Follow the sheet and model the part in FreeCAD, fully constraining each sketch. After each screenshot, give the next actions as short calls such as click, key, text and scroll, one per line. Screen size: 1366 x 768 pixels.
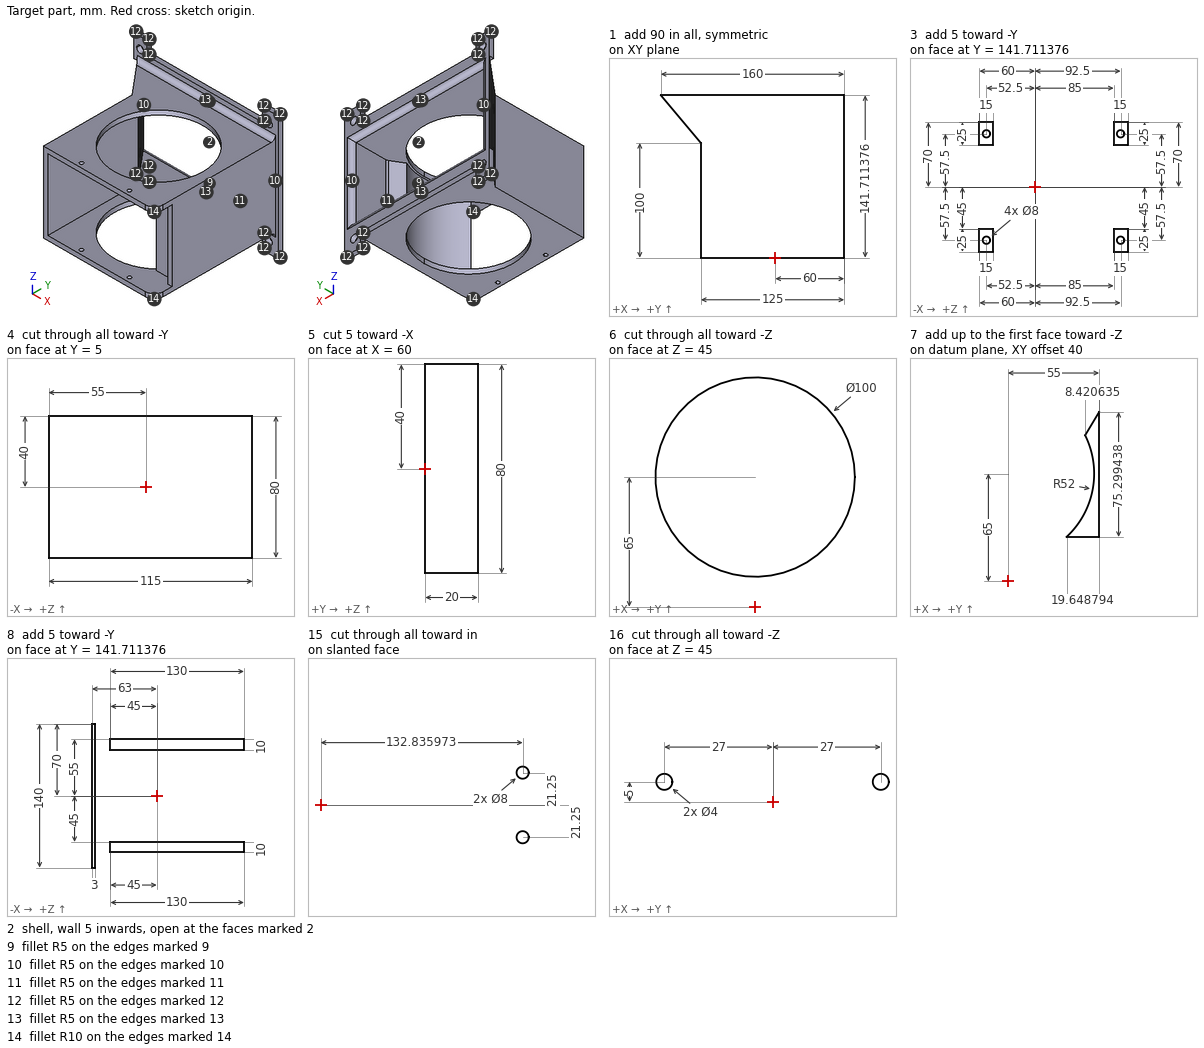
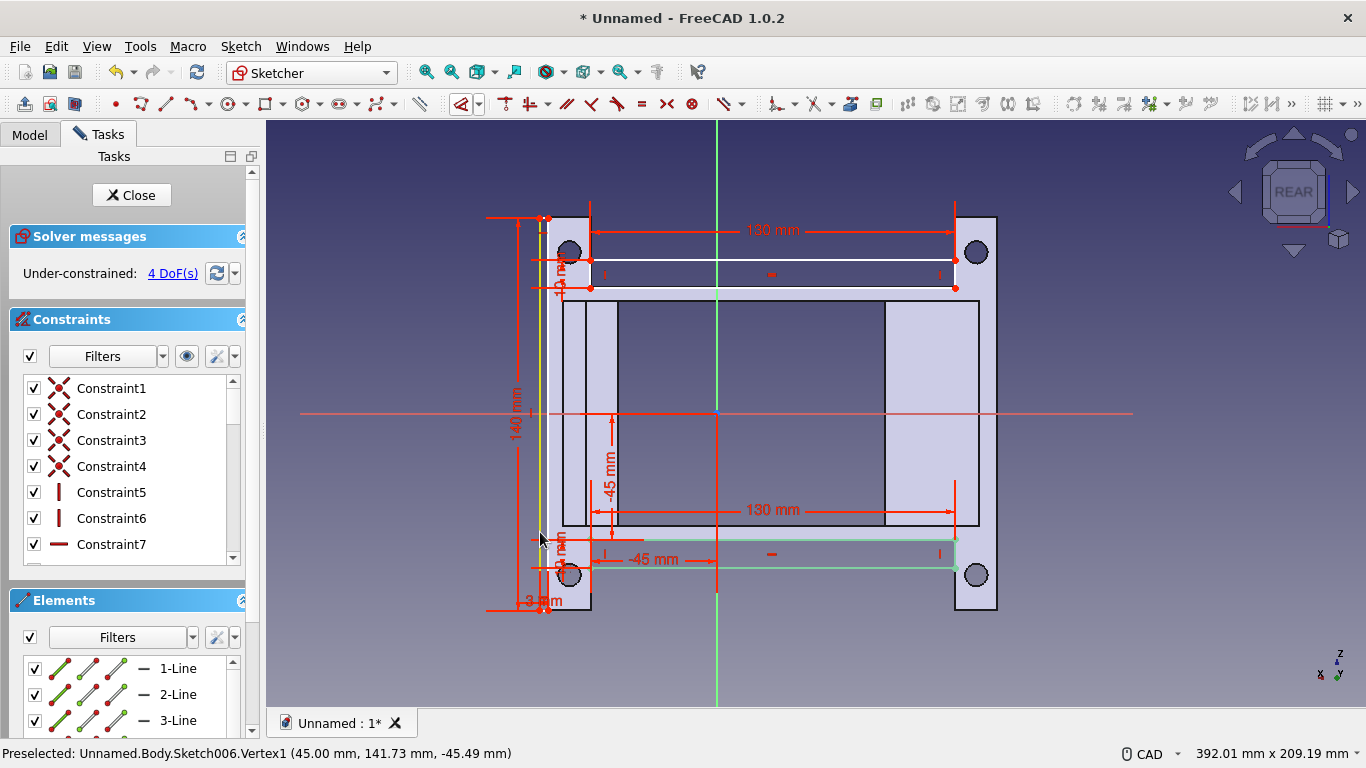
click(590, 260)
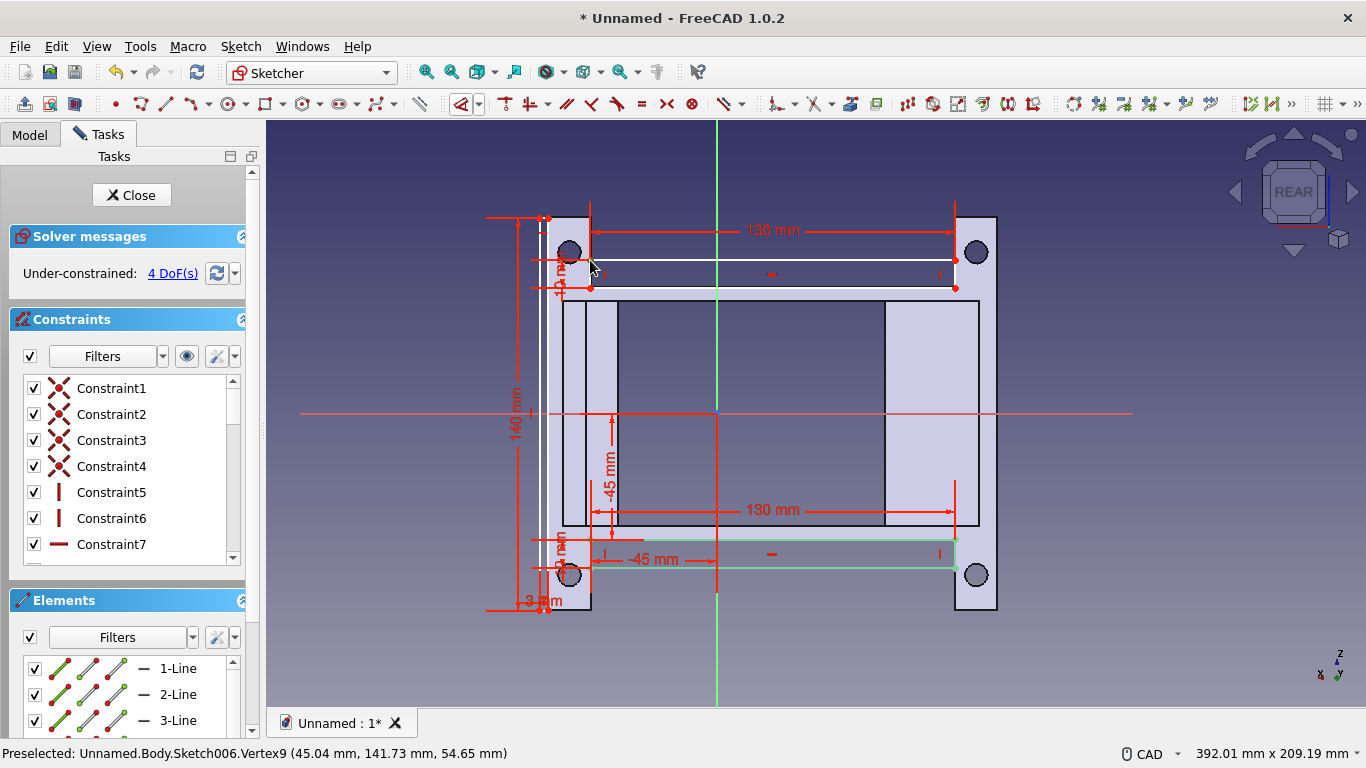
key(l)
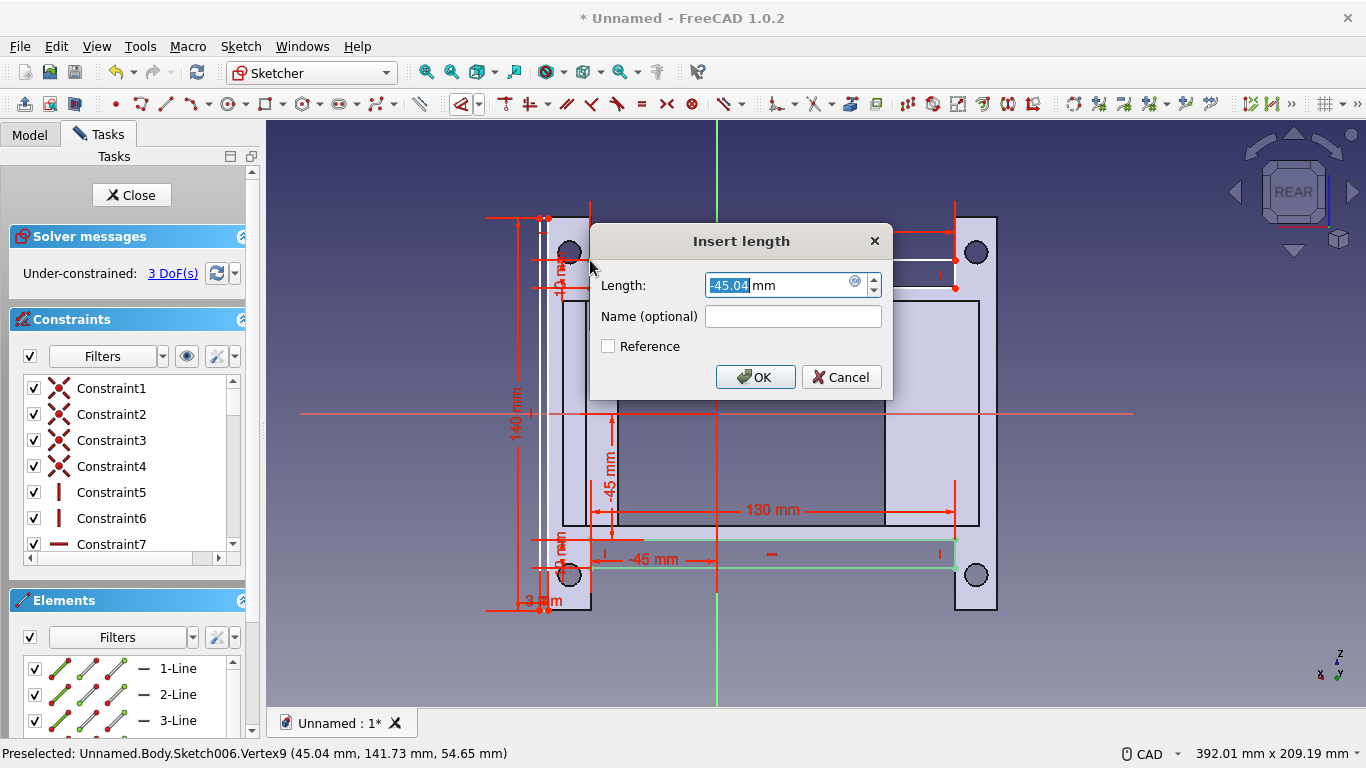
text(-45)
key(Return)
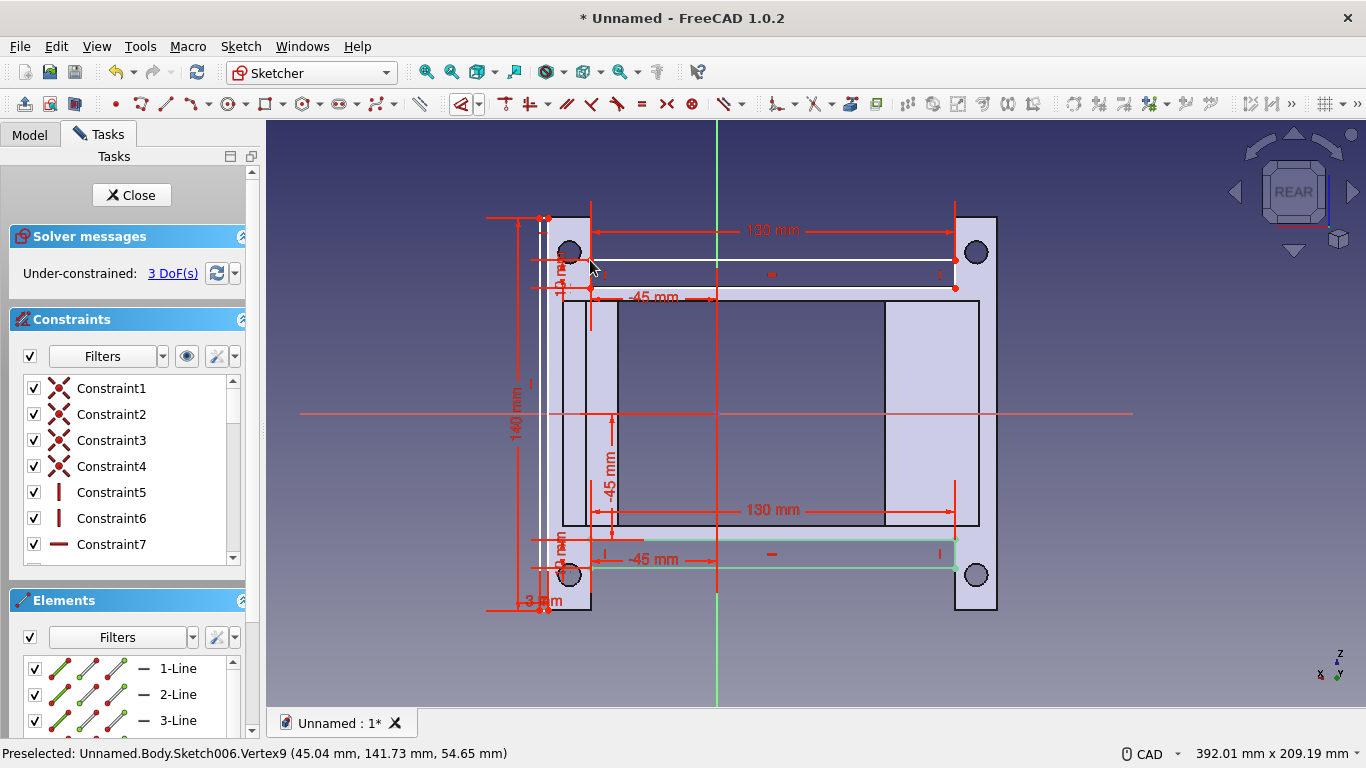
click(591, 260)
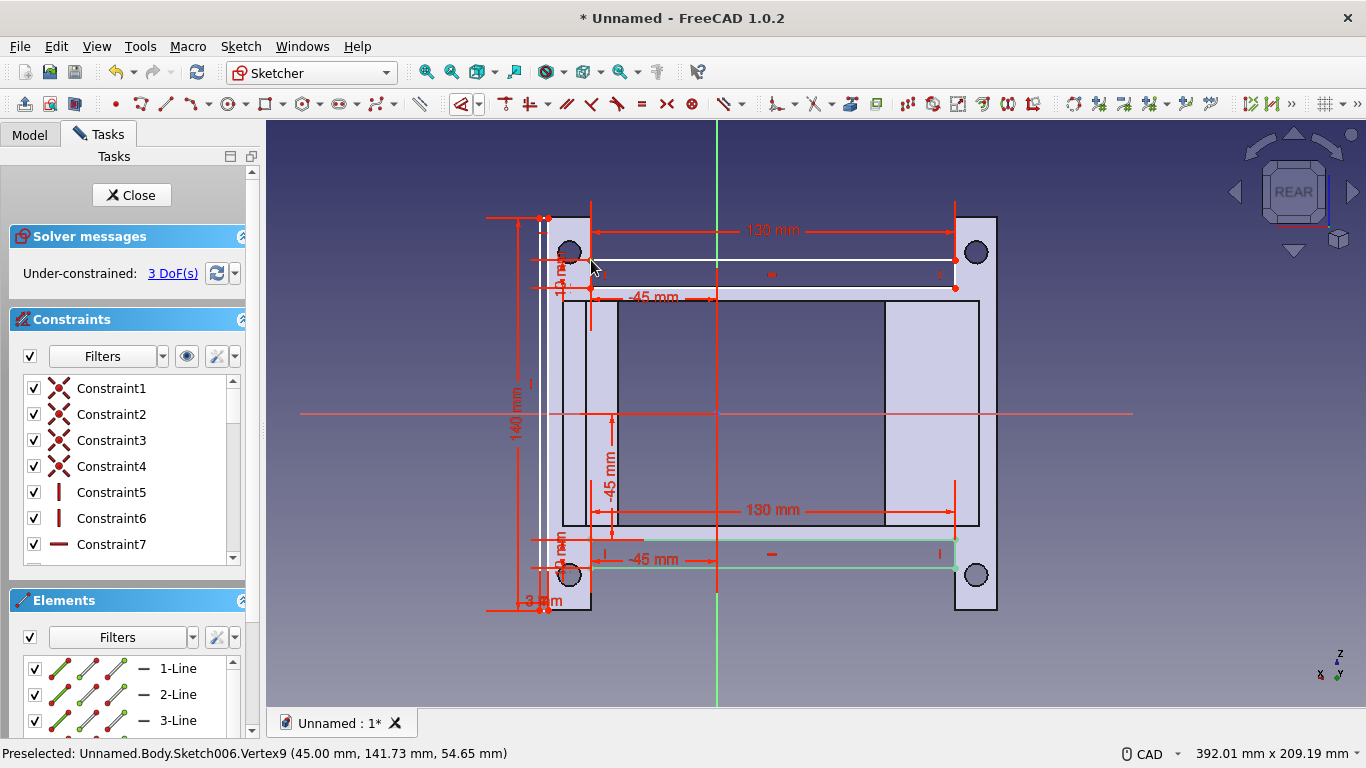
key(i)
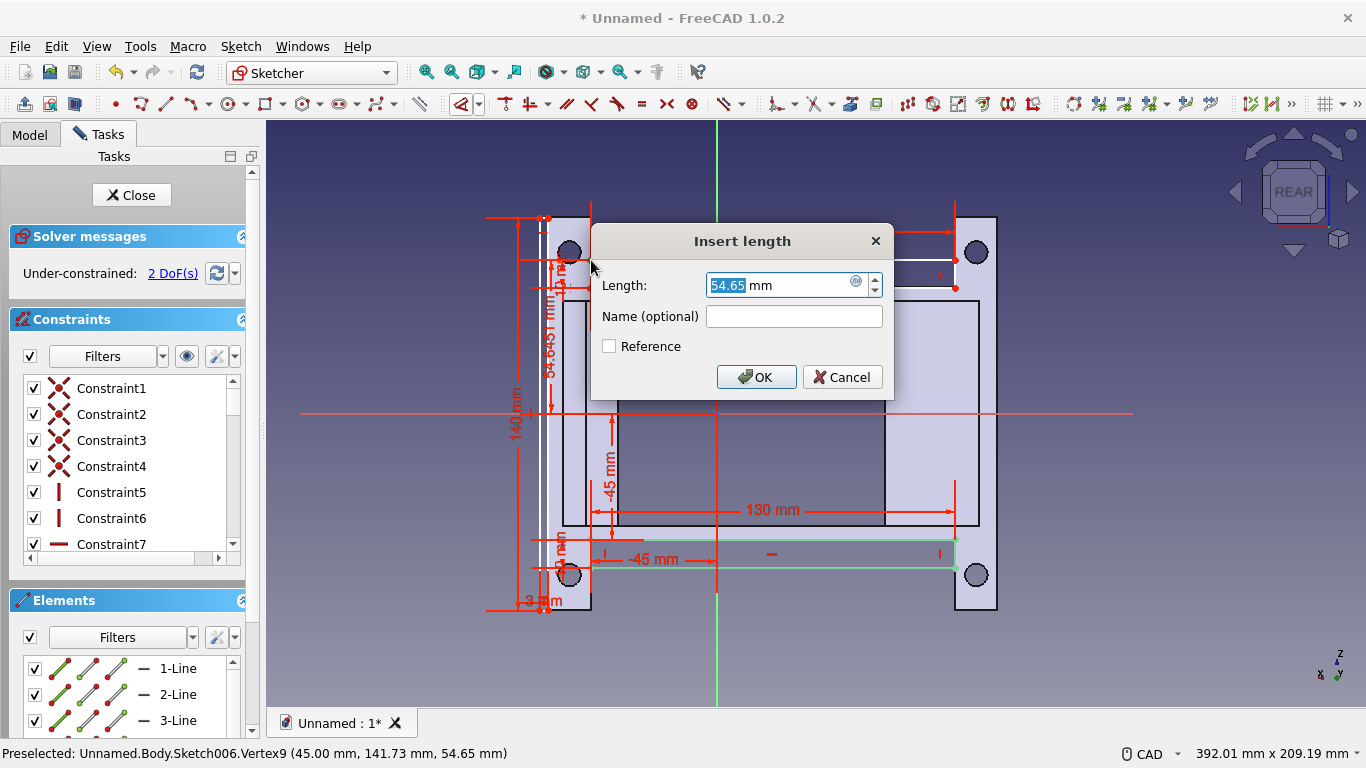
text(55)
key(Return)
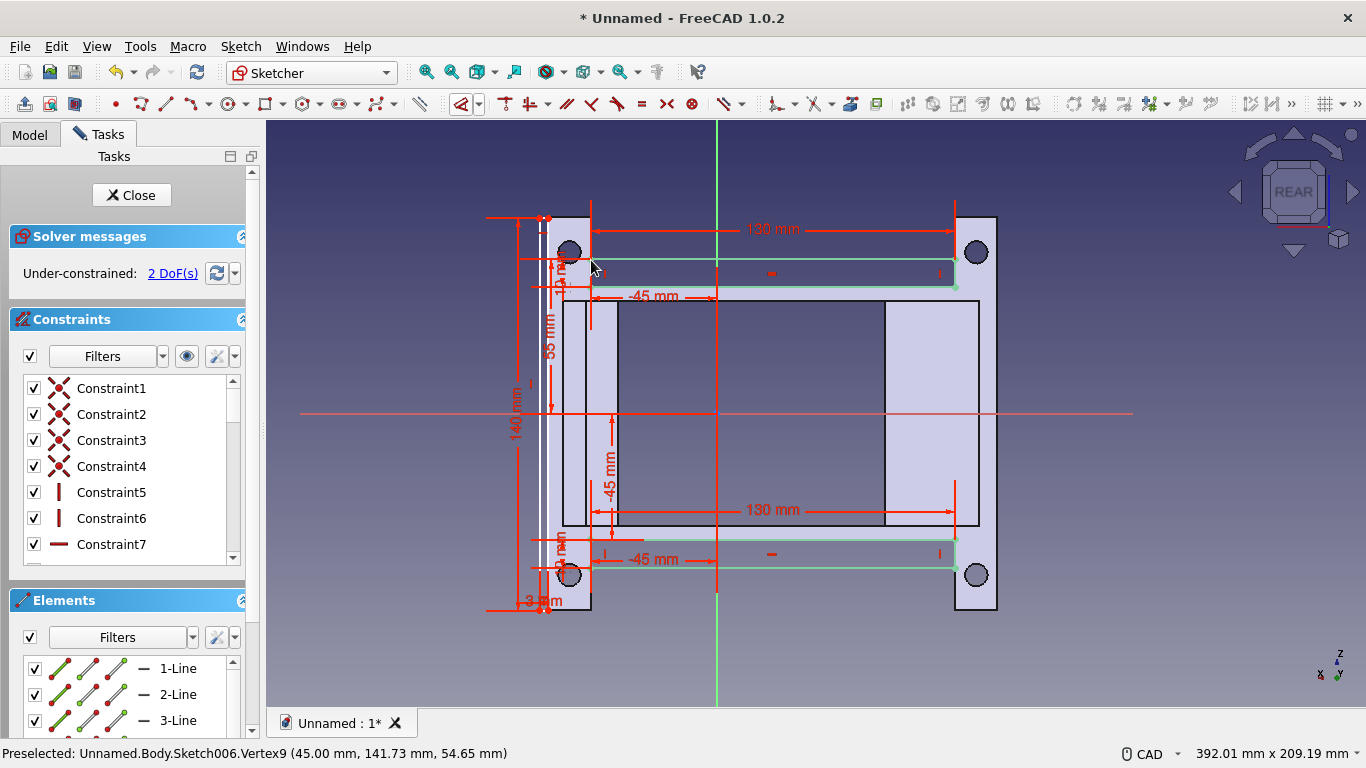
scroll(540, 218, up, 2)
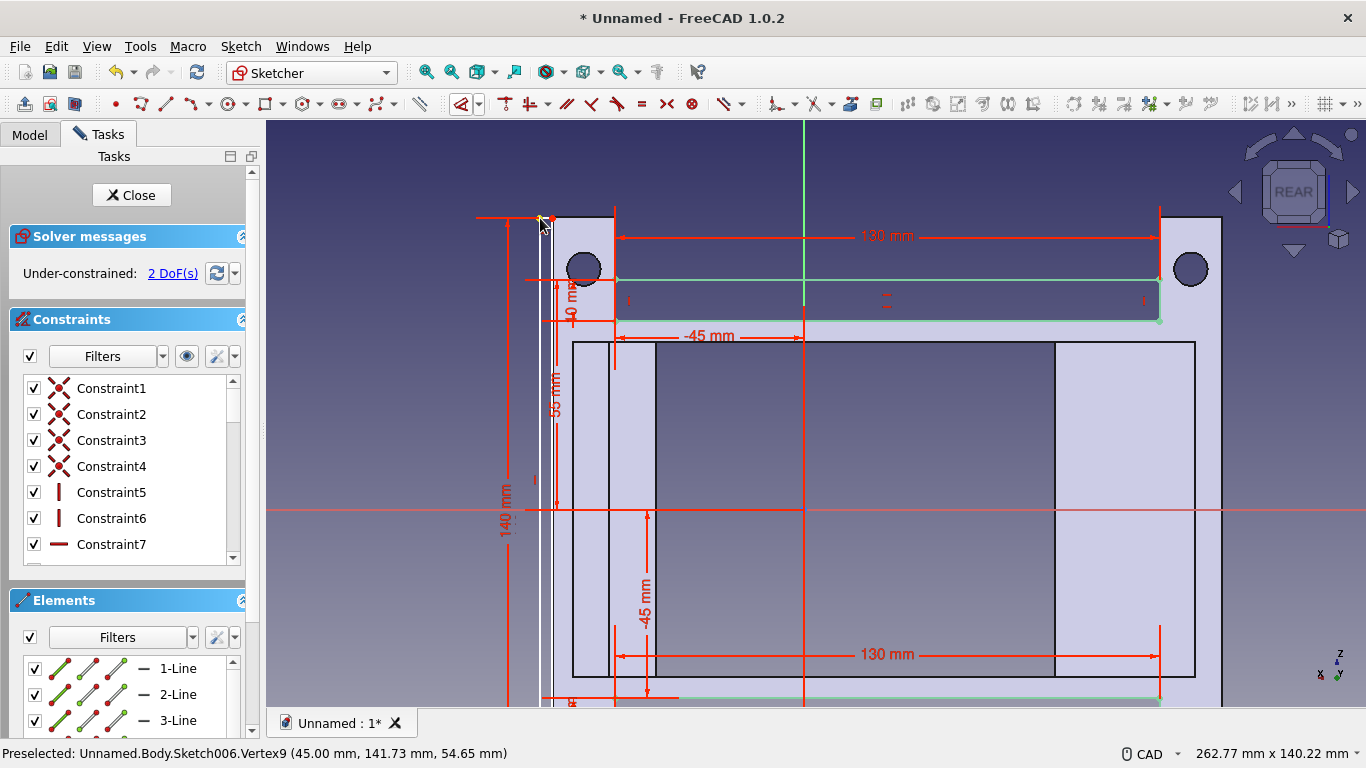
click(540, 218)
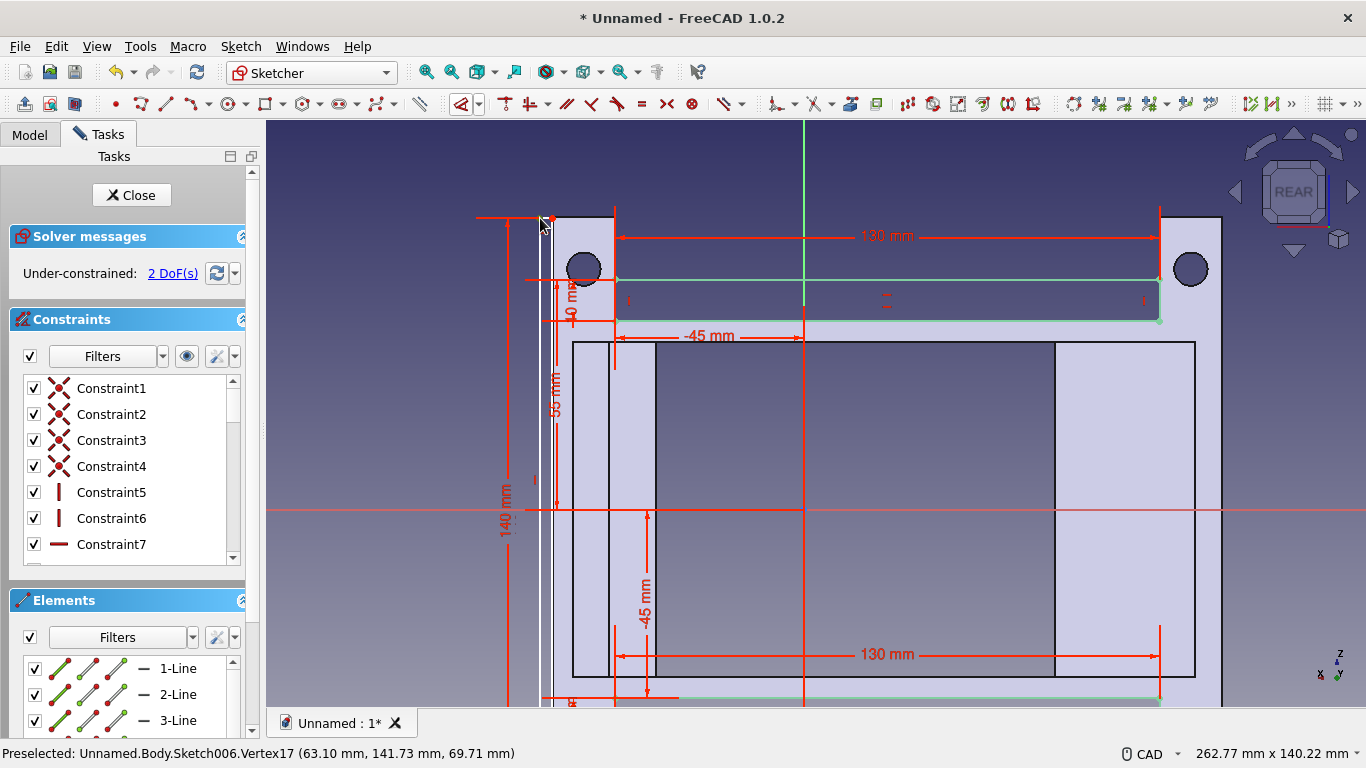
key(l)